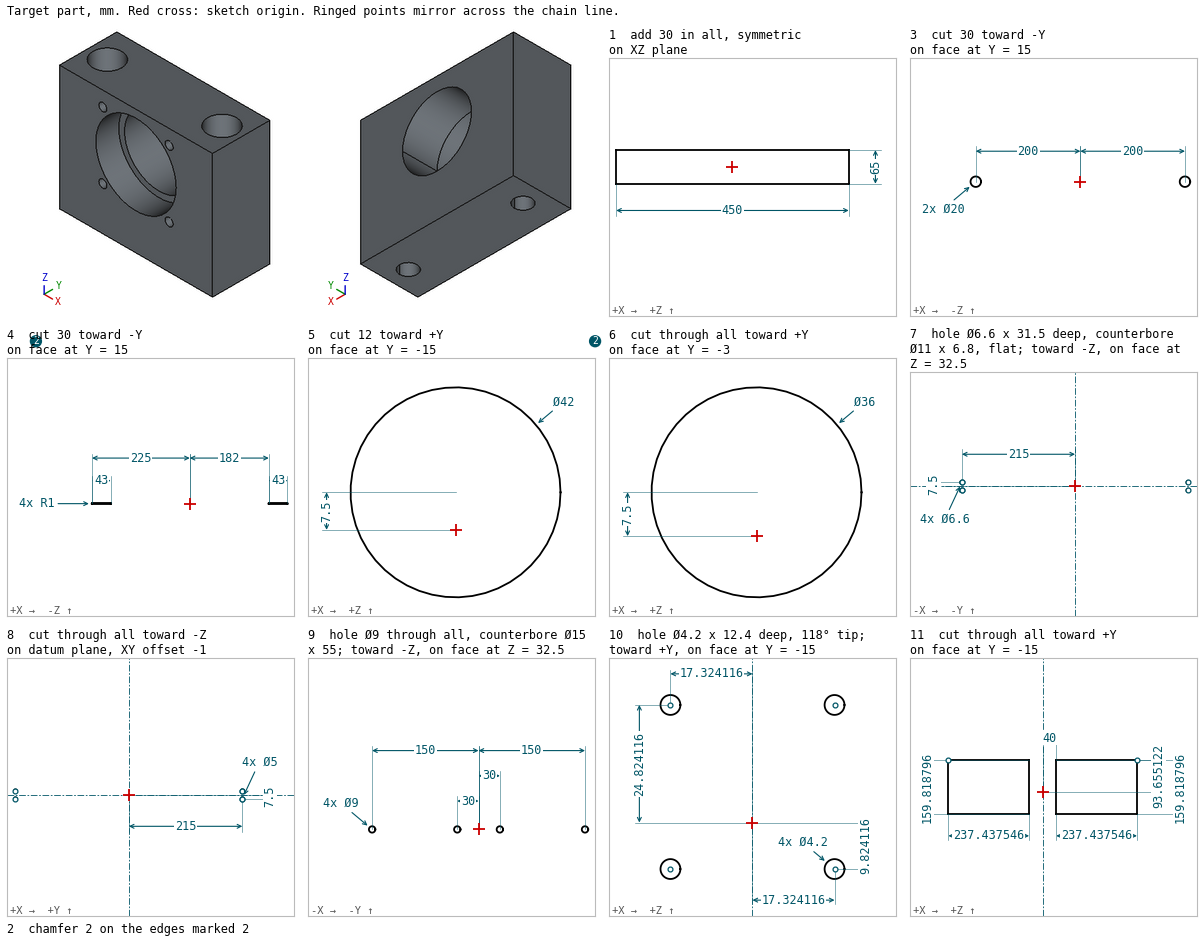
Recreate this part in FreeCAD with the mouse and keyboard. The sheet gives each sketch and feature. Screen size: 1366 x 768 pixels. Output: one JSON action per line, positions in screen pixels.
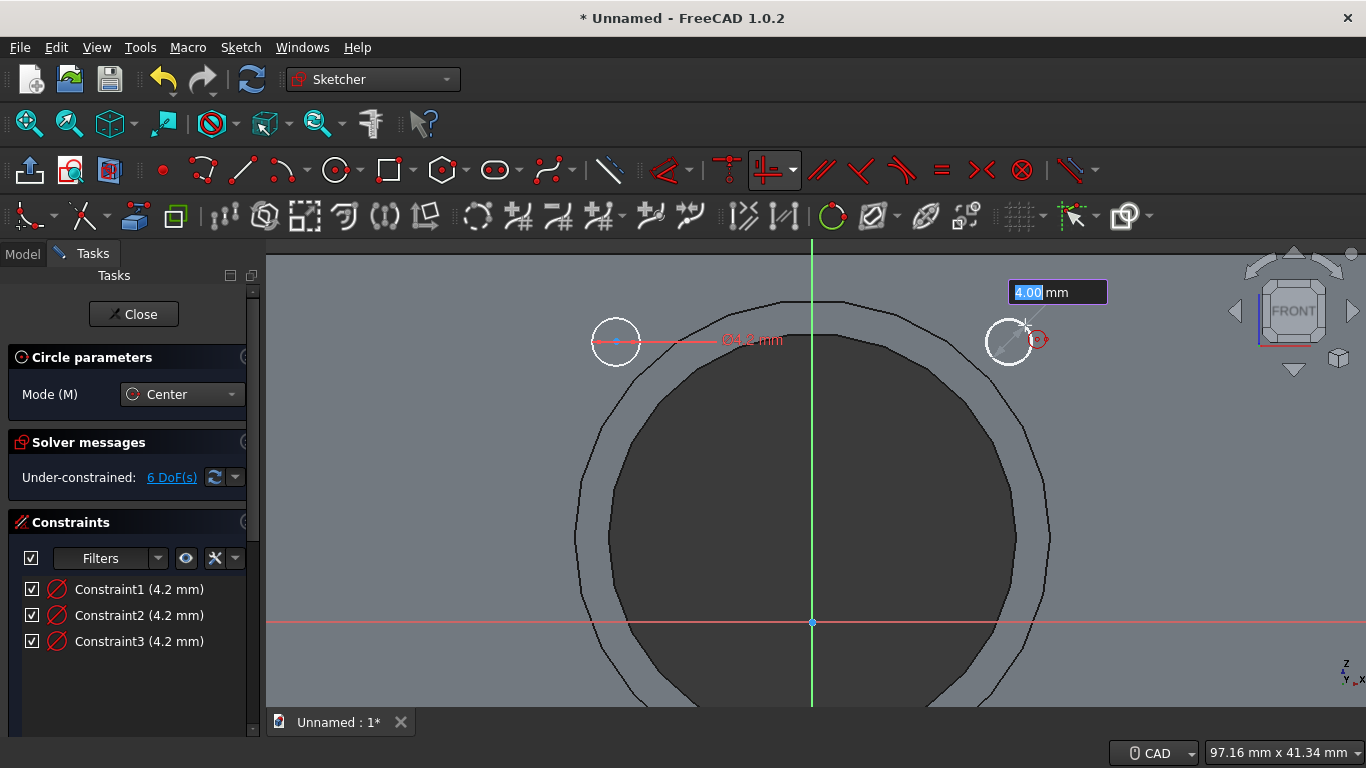
{"action": "type", "text": "4.2"}
{"action": "key", "text": "Return"}
{"action": "key", "text": "Escape"}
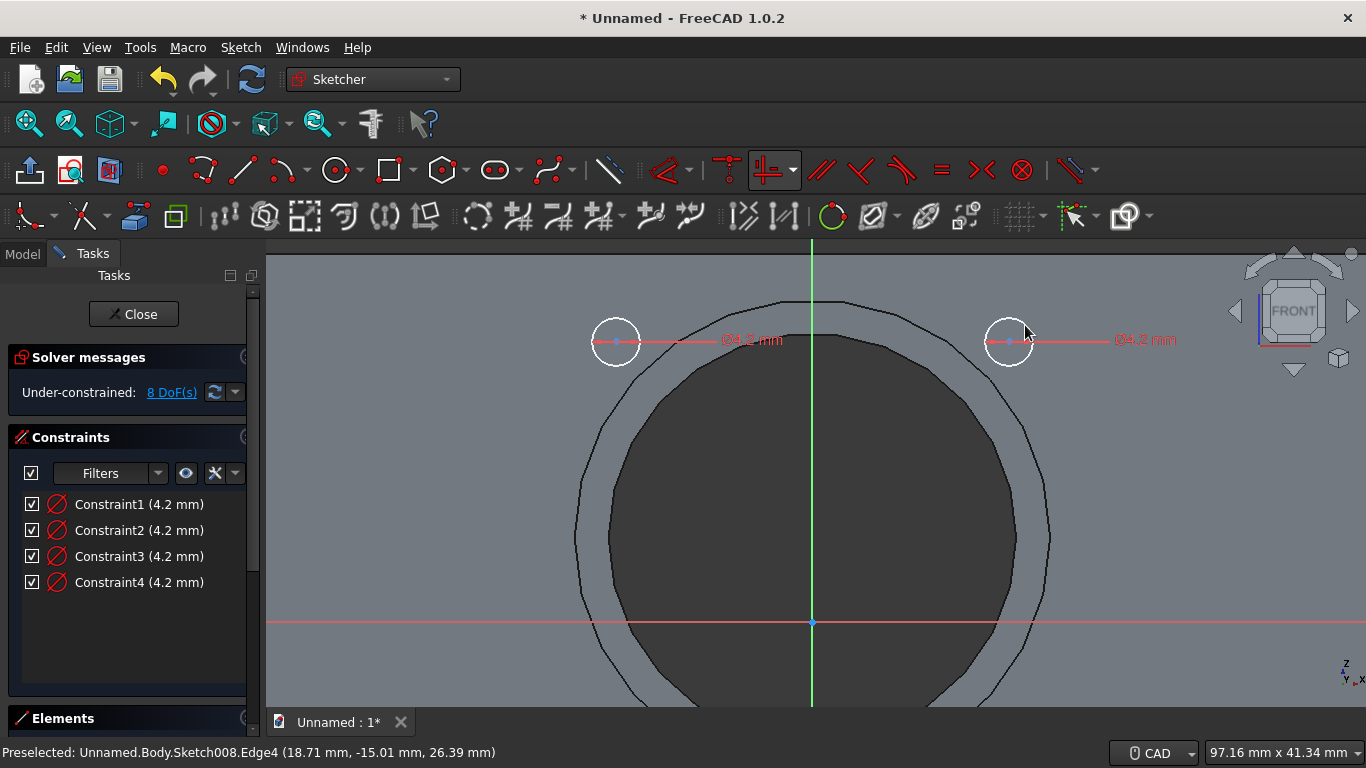
{"action": "scroll", "coordinate": [616, 342], "scroll_direction": "down", "scroll_amount": 2}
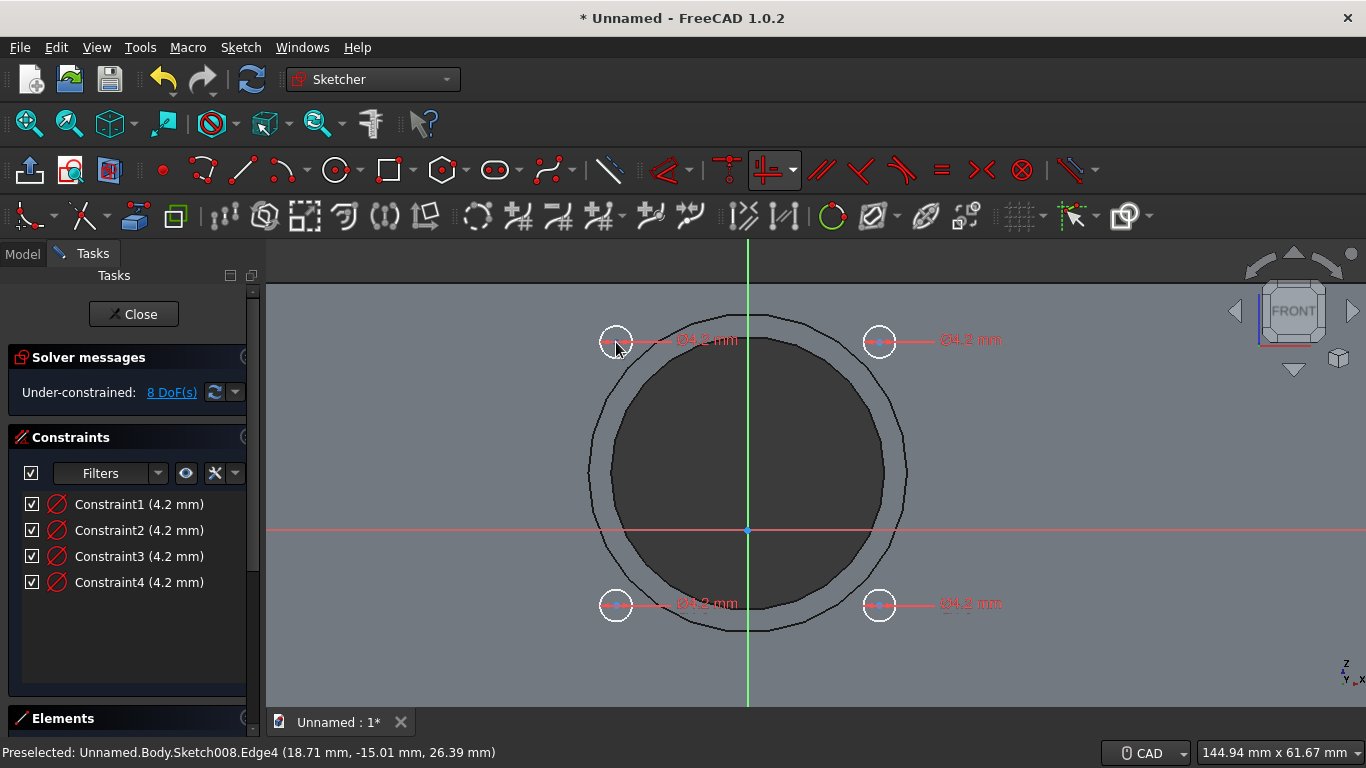
{"action": "left_click", "coordinate": [879, 606]}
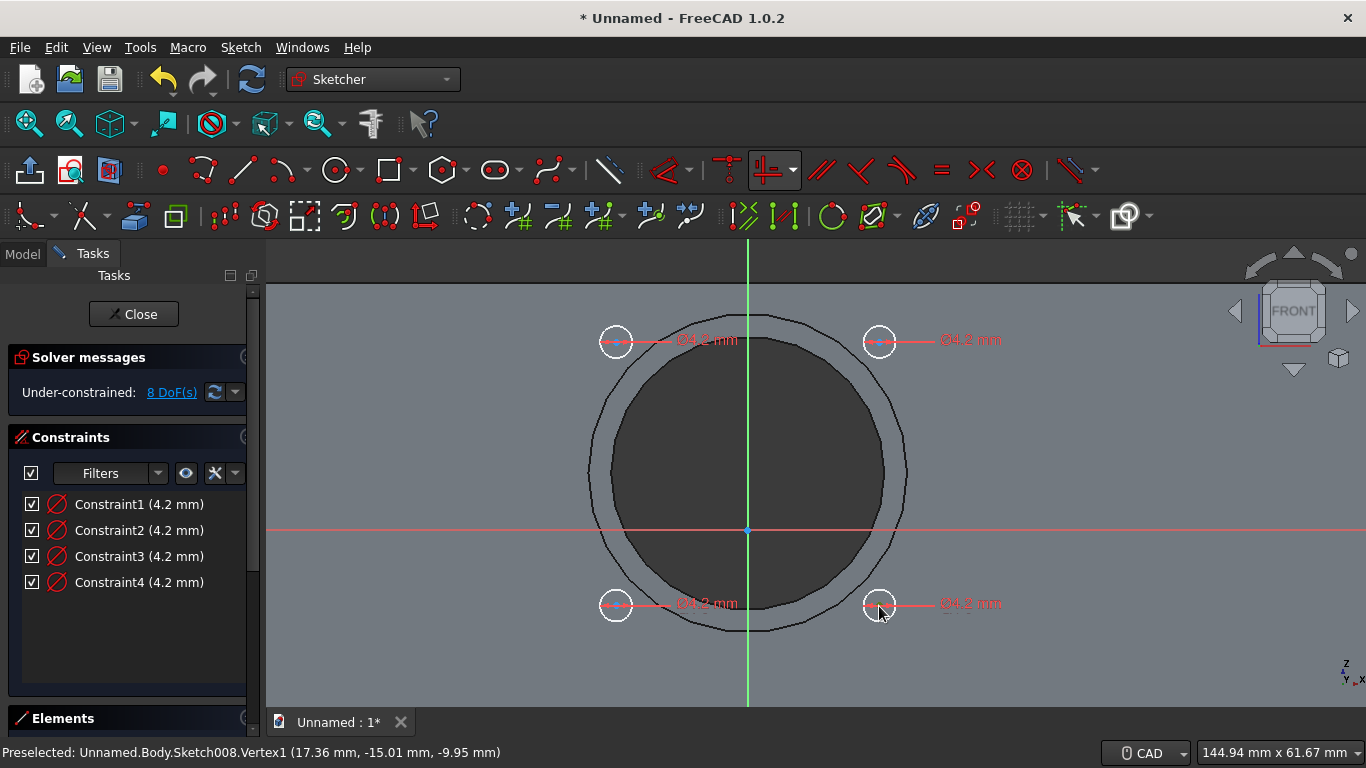
{"action": "left_click", "coordinate": [616, 606]}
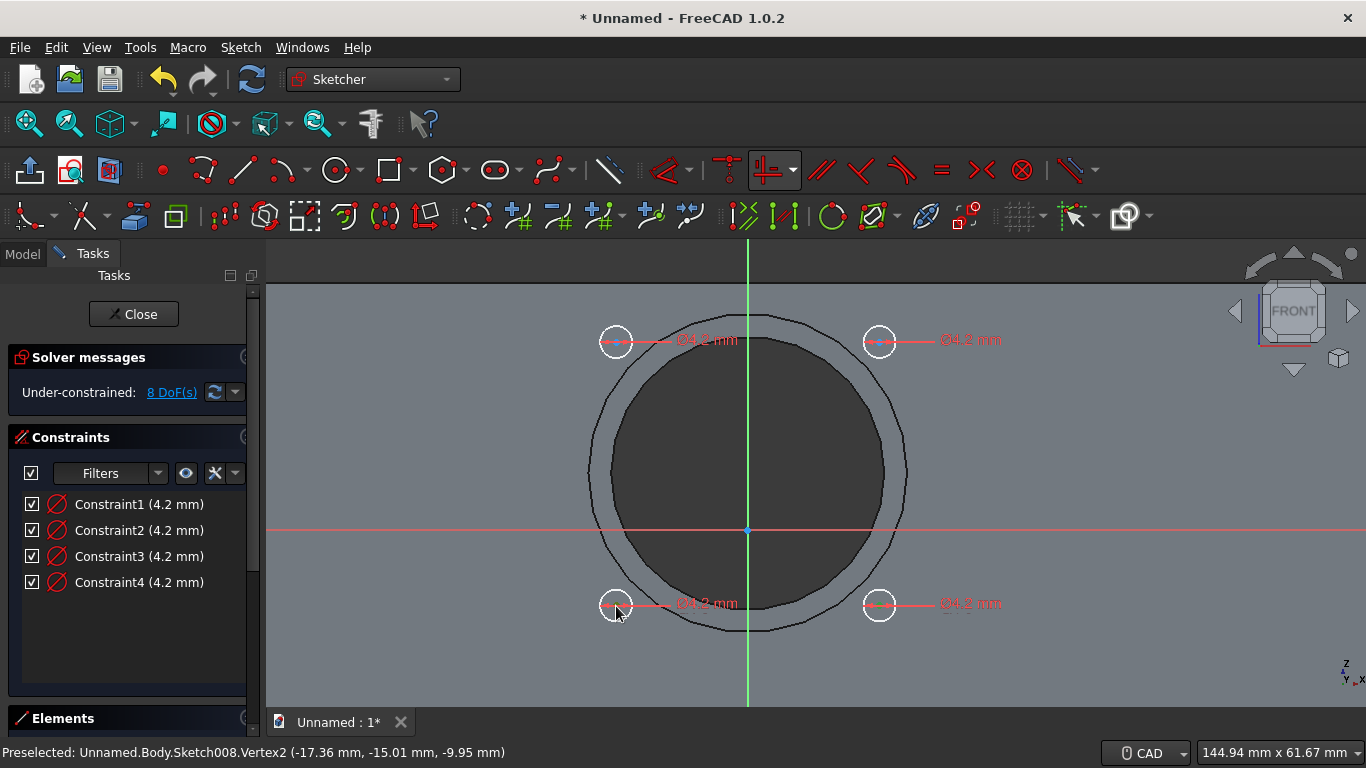
{"action": "left_click", "coordinate": [748, 650]}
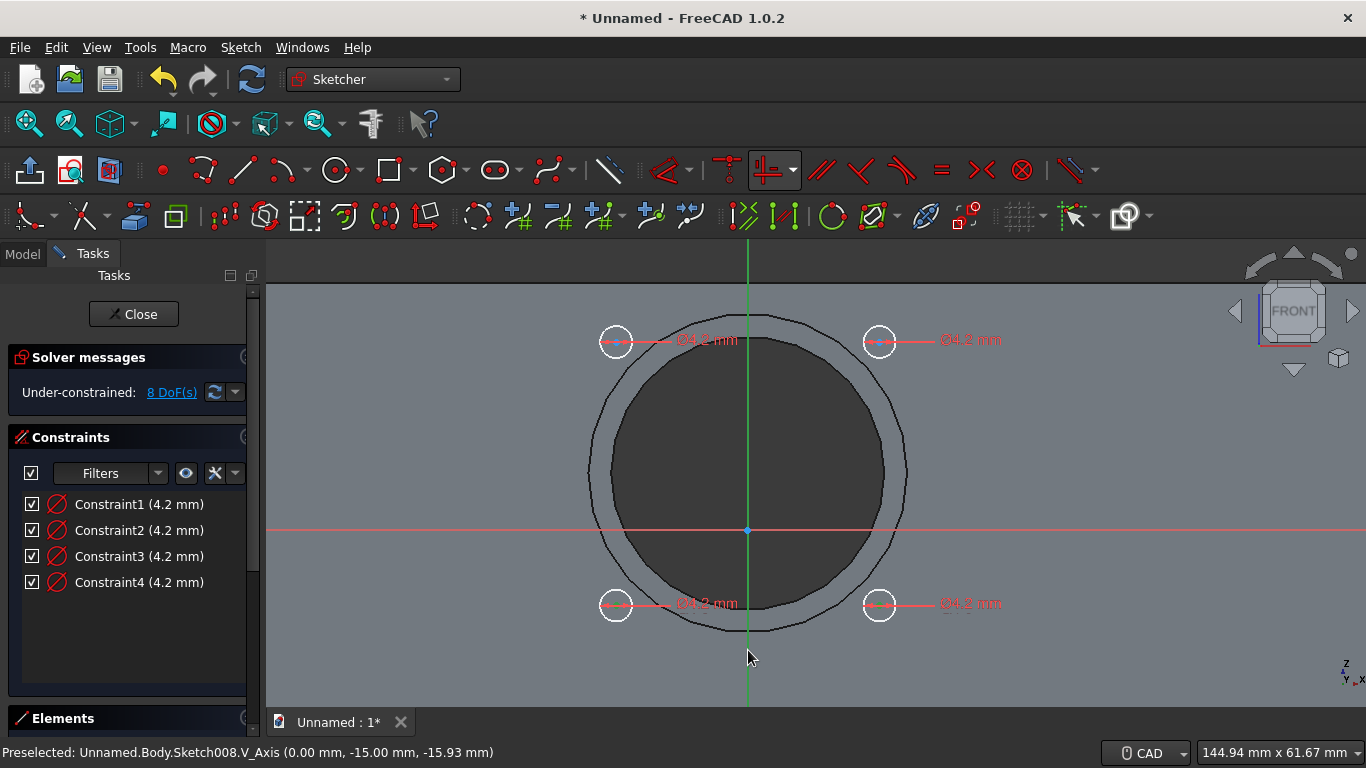
{"action": "key", "text": "s"}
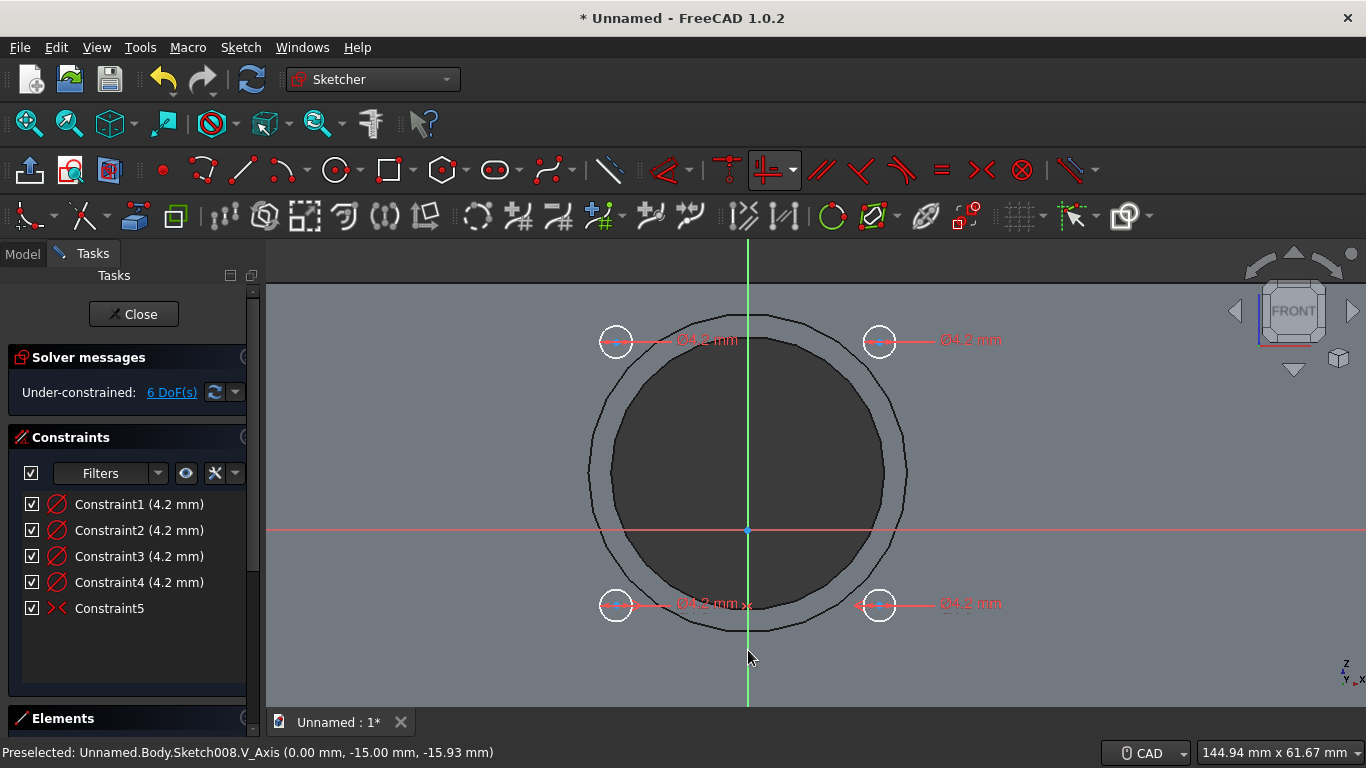
{"action": "left_click", "coordinate": [616, 342]}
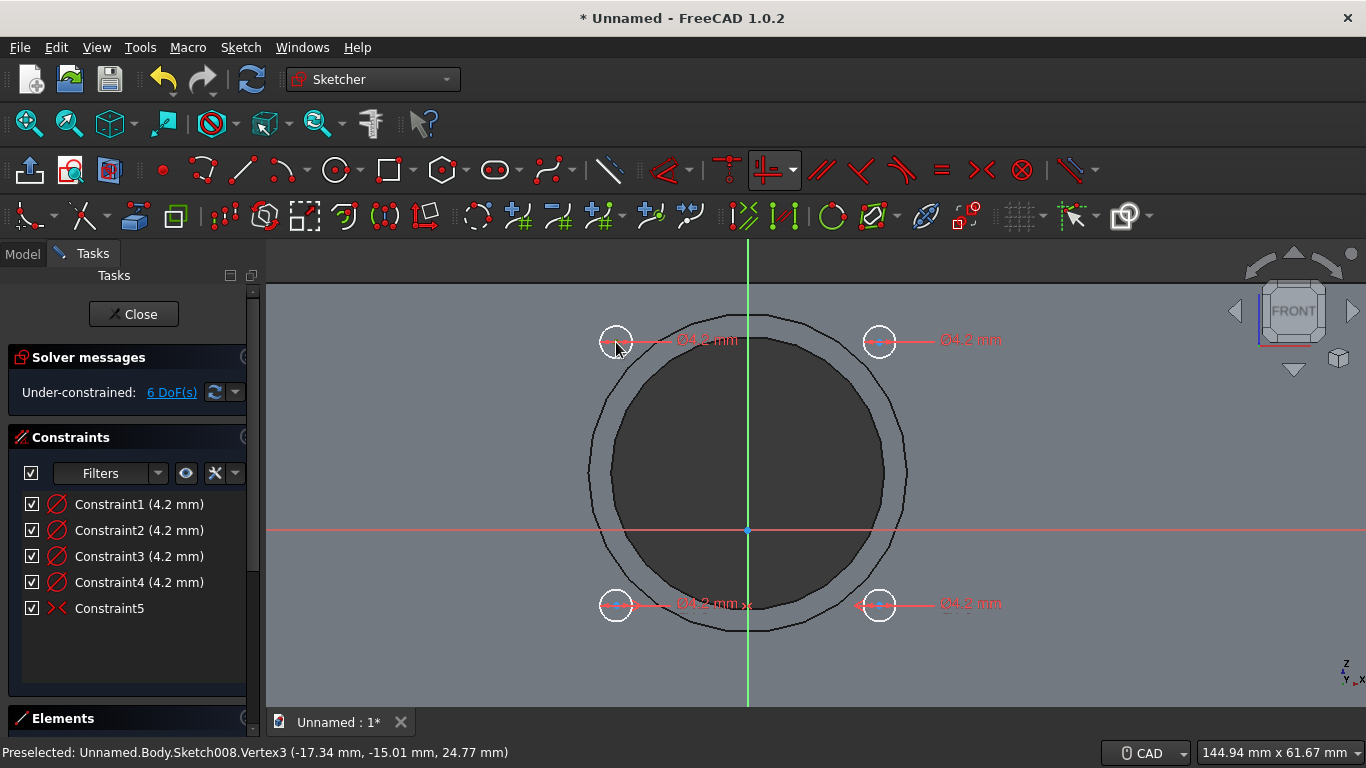
{"action": "left_click", "coordinate": [880, 342]}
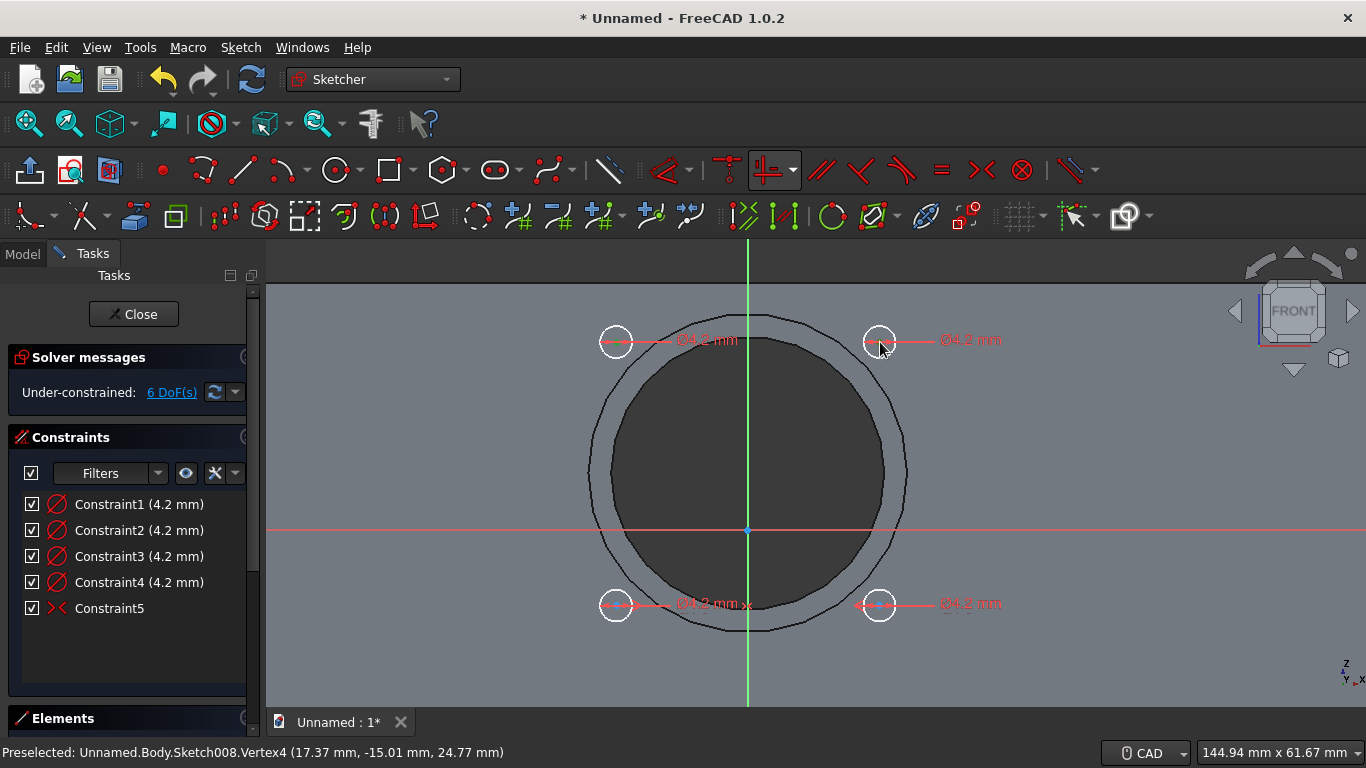
{"action": "left_click", "coordinate": [748, 650]}